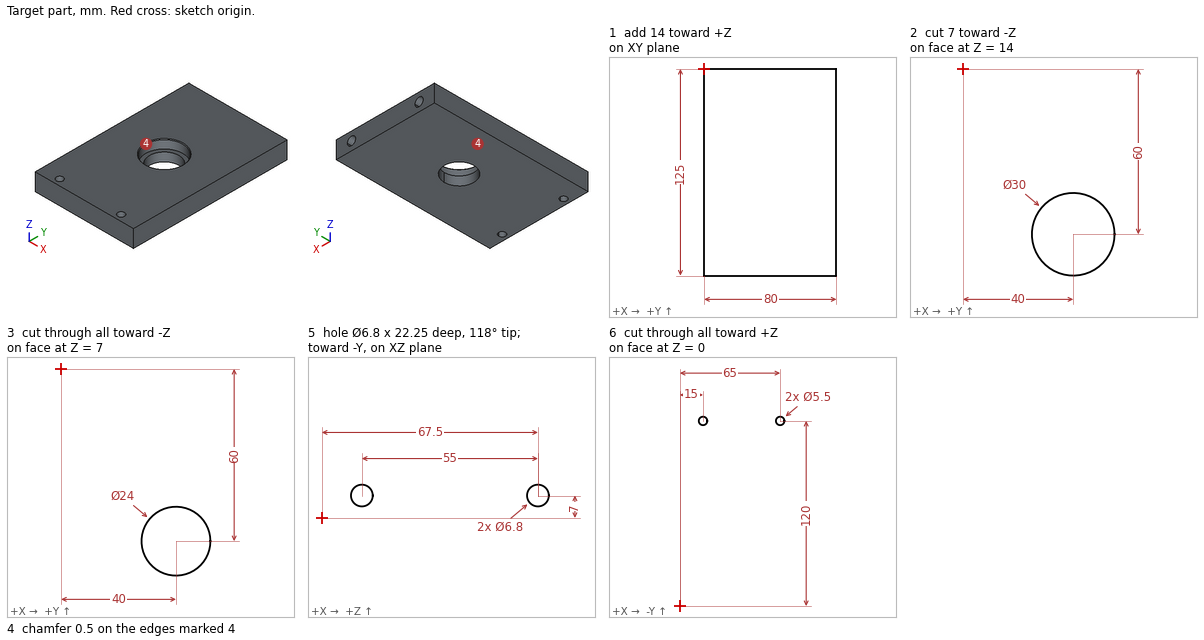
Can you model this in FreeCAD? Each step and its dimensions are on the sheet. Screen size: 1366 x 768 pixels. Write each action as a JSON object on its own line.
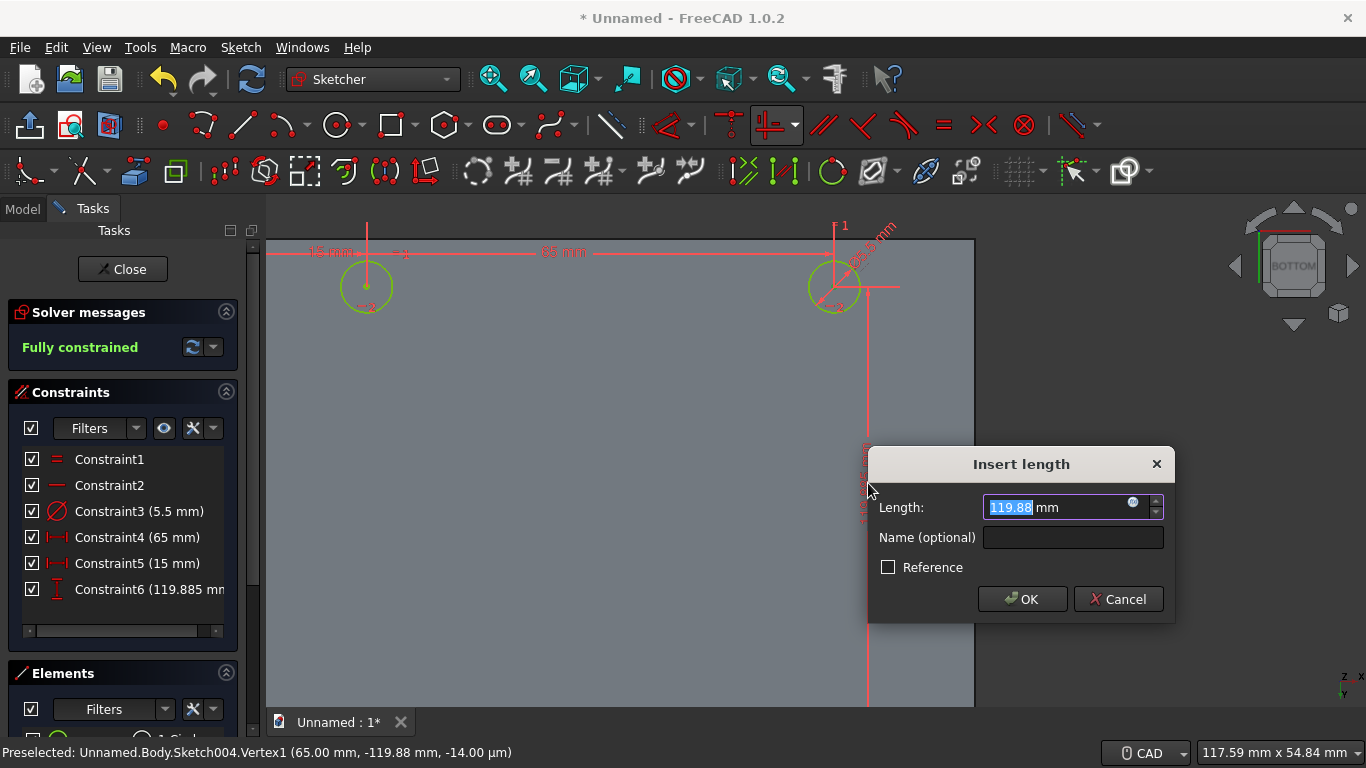
{"action": "type", "text": "120"}
{"action": "key", "text": "Return"}
{"action": "key", "text": "Escape"}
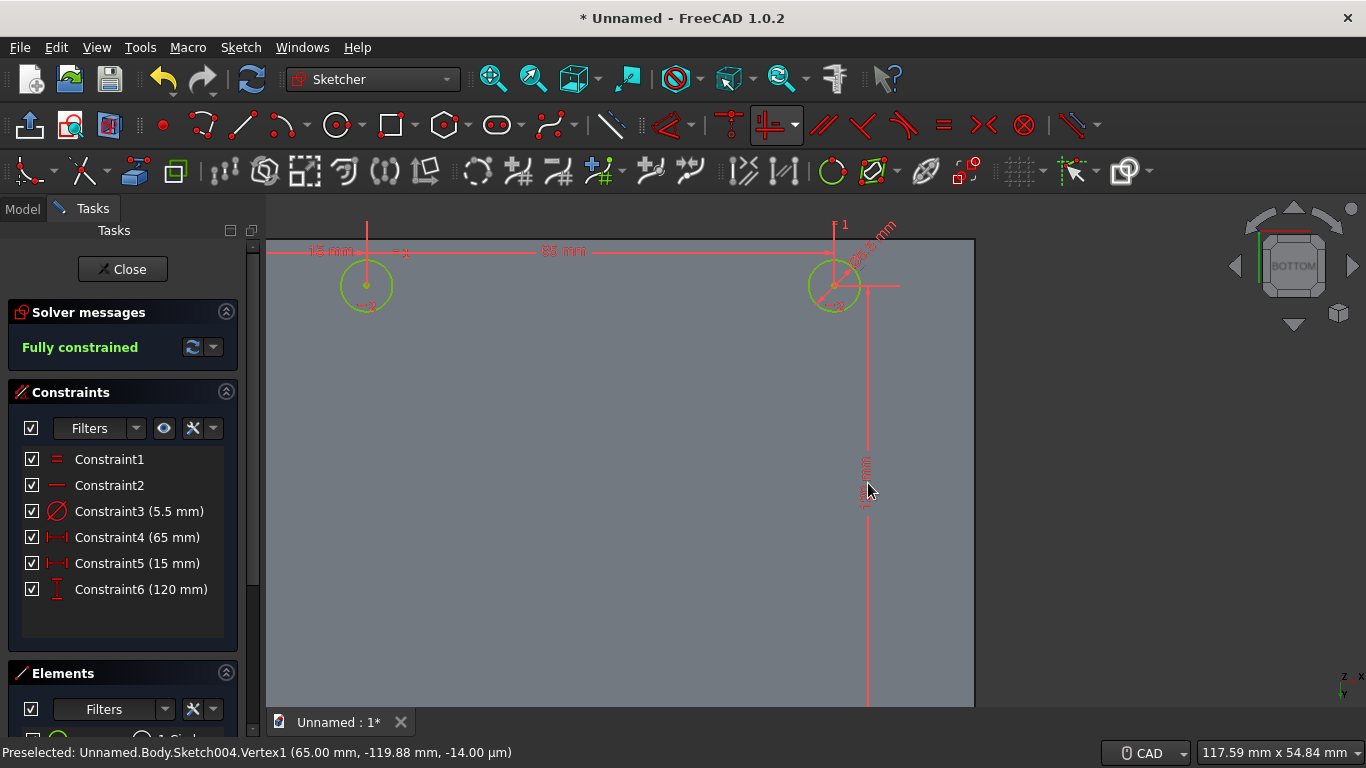
{"action": "left_click", "coordinate": [123, 269]}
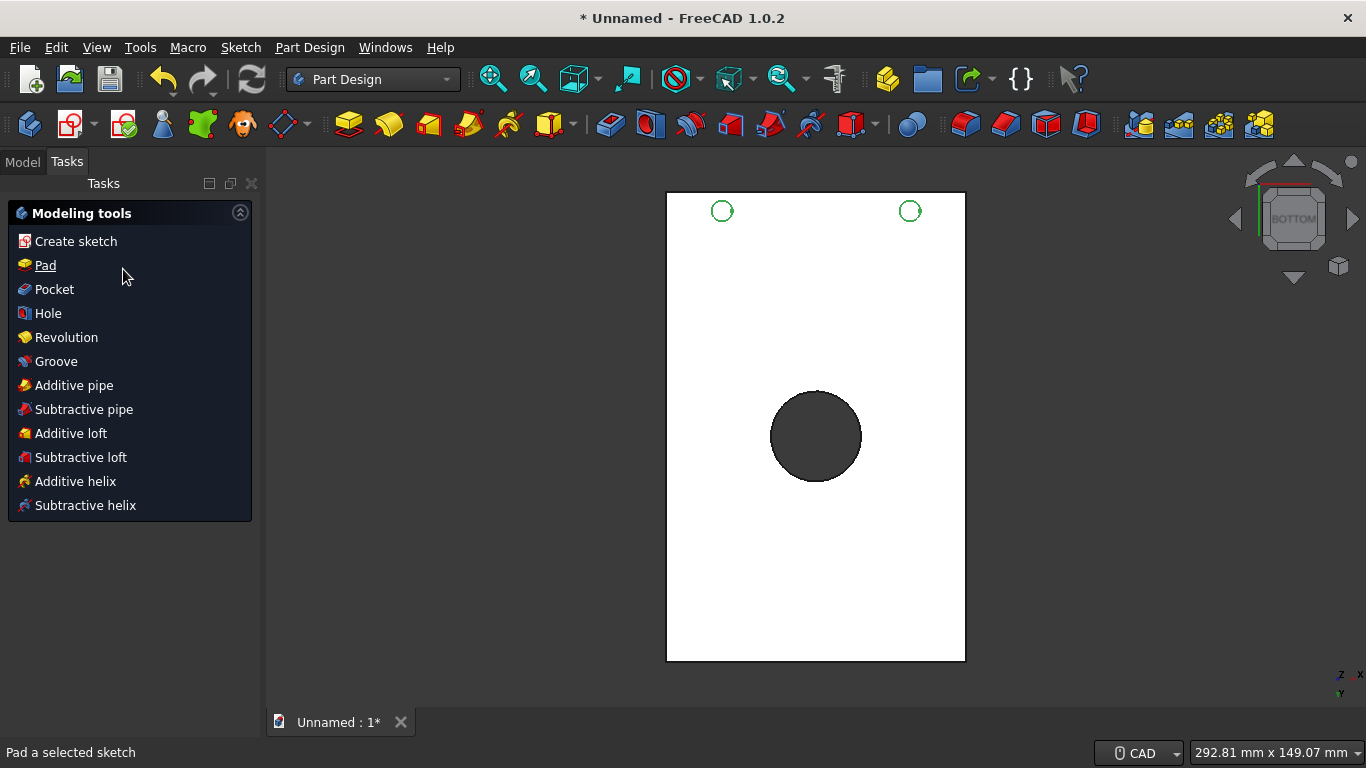
{"action": "left_click", "coordinate": [612, 124]}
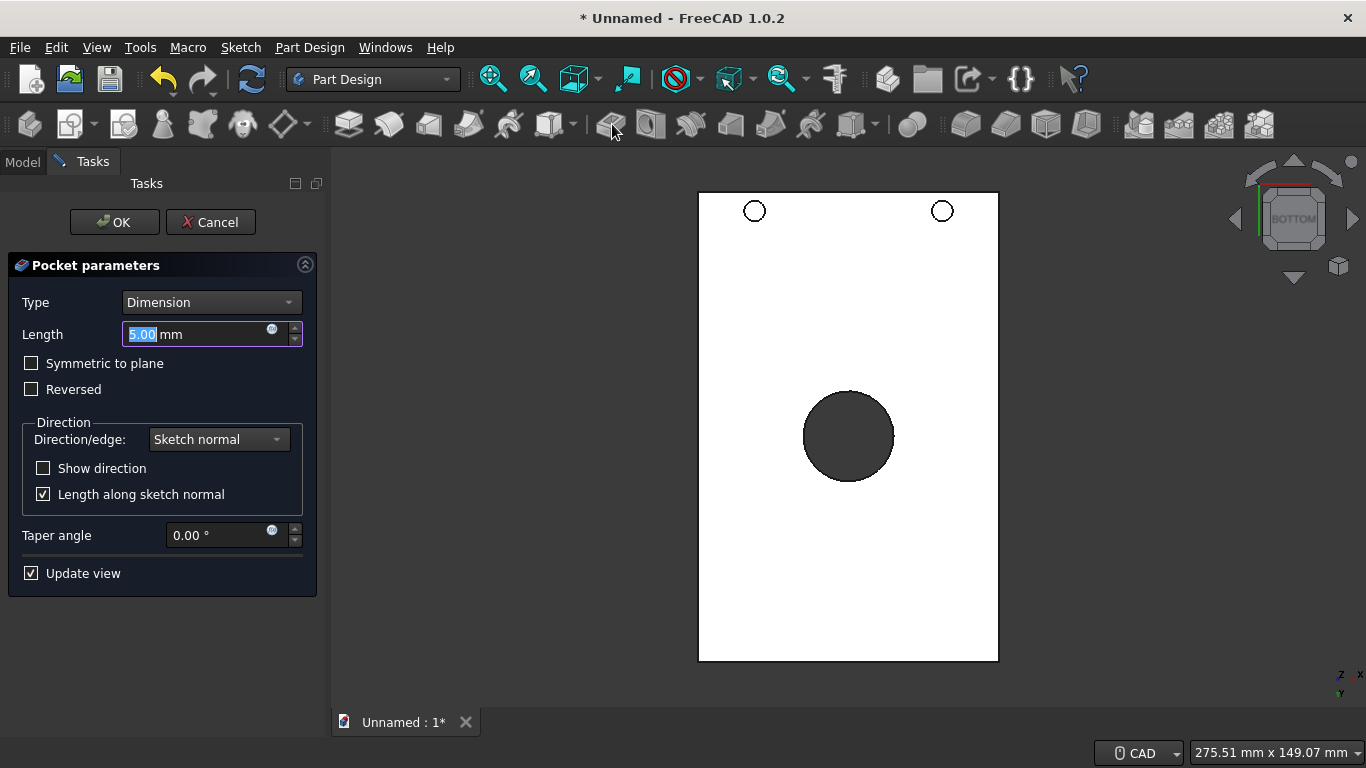
{"action": "left_click", "coordinate": [212, 302]}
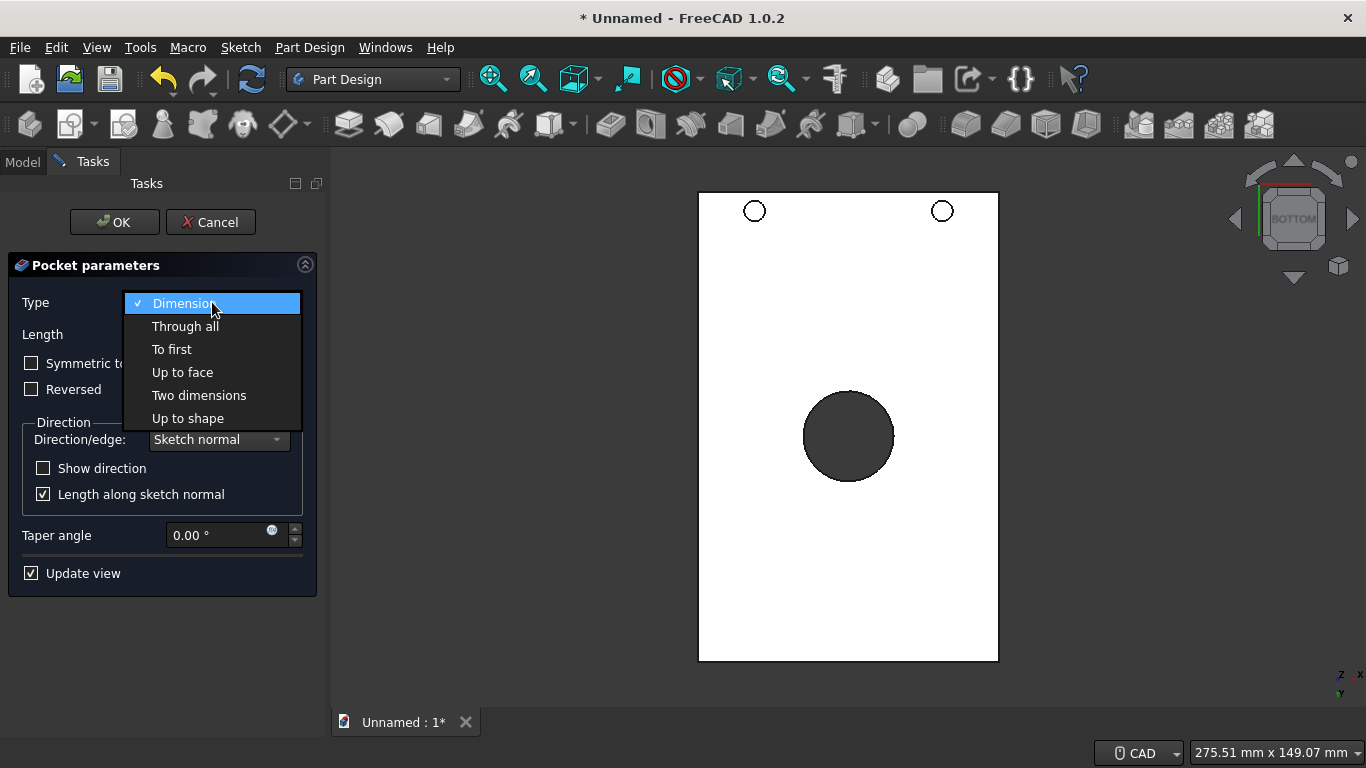
{"action": "left_click", "coordinate": [212, 326]}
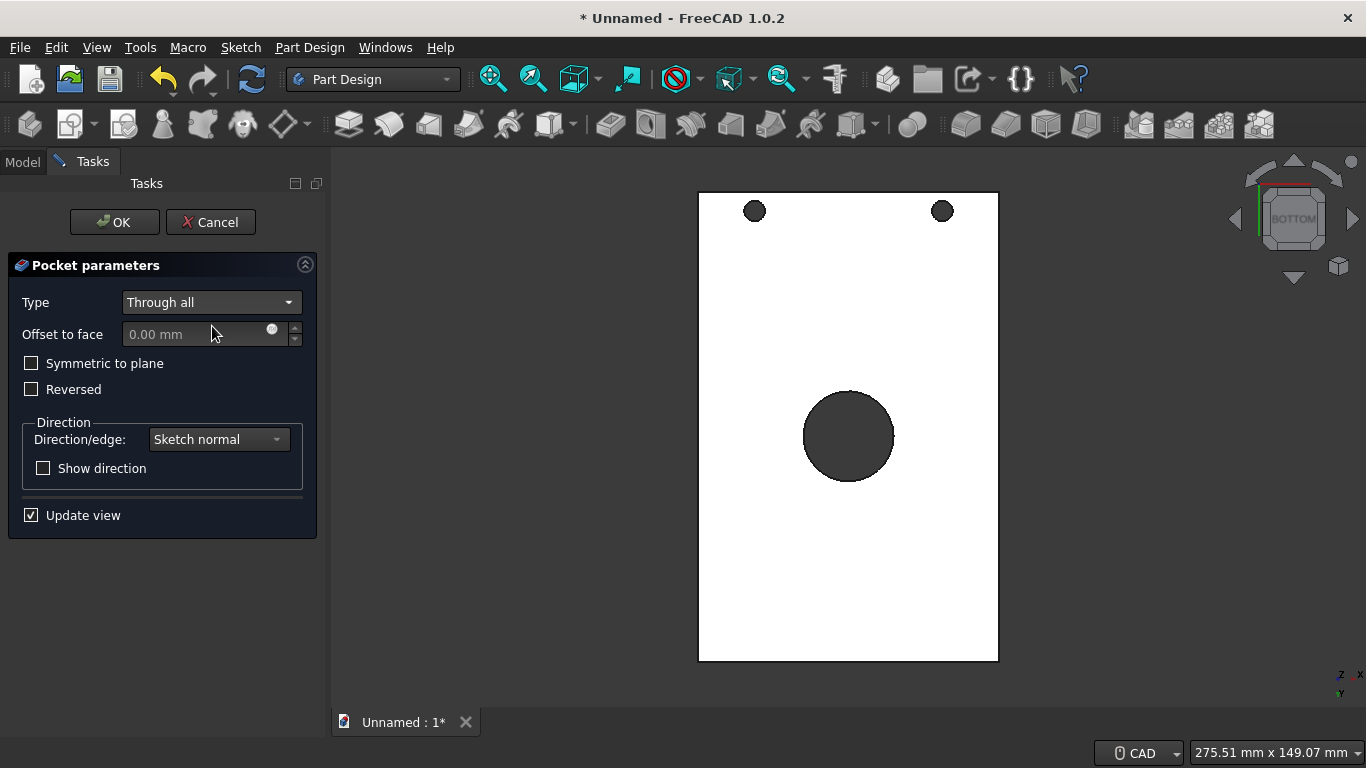
{"action": "left_click", "coordinate": [115, 222]}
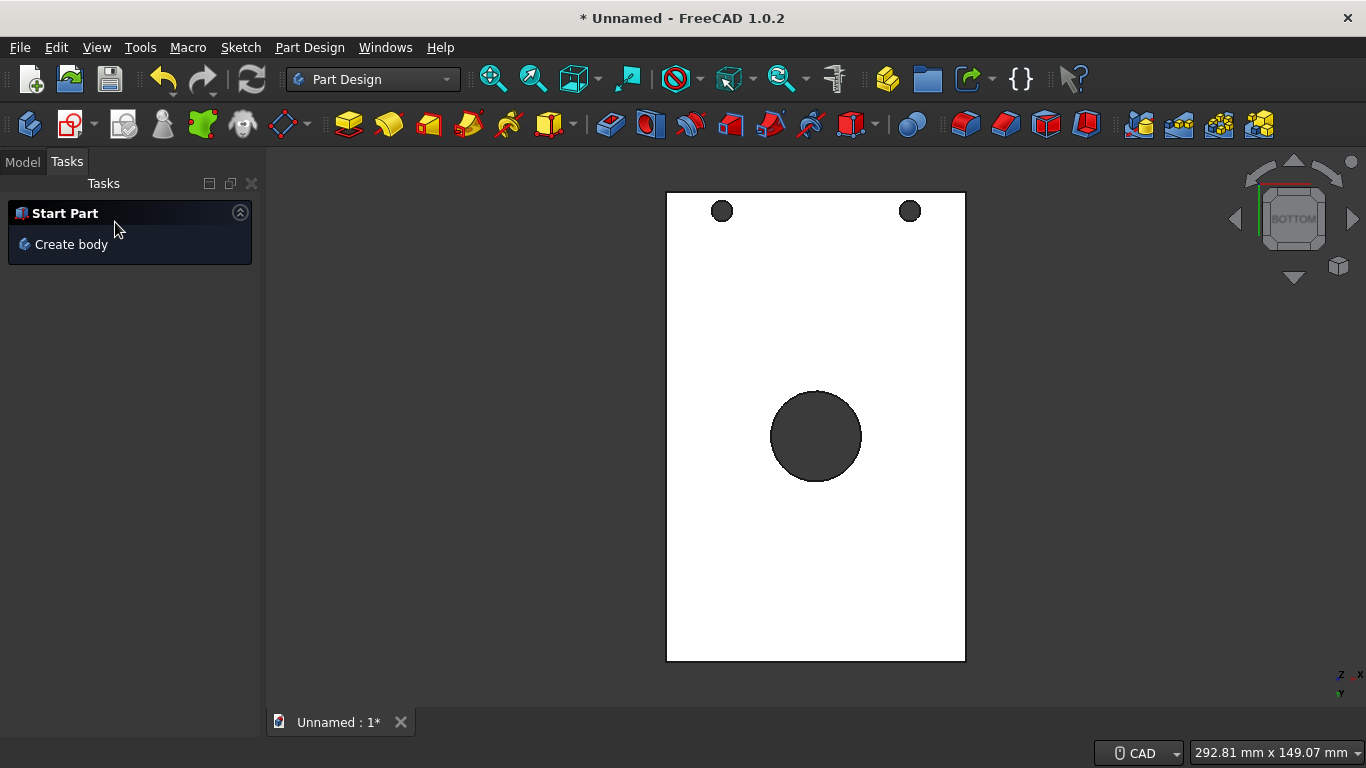
{"action": "key", "text": "0"}